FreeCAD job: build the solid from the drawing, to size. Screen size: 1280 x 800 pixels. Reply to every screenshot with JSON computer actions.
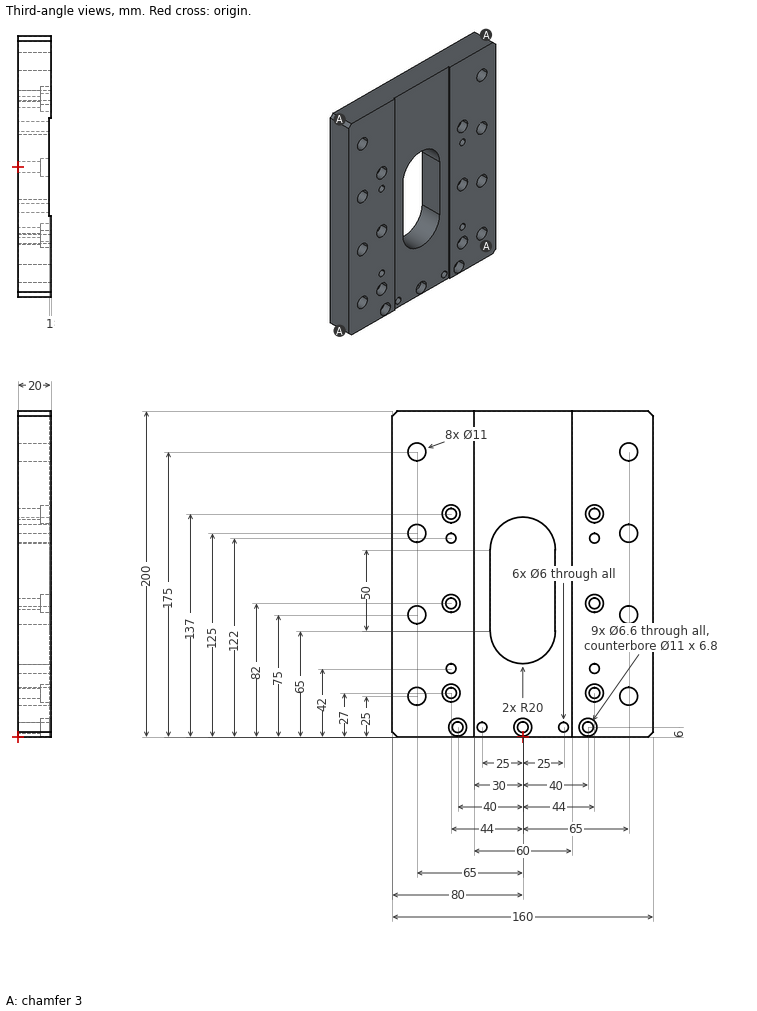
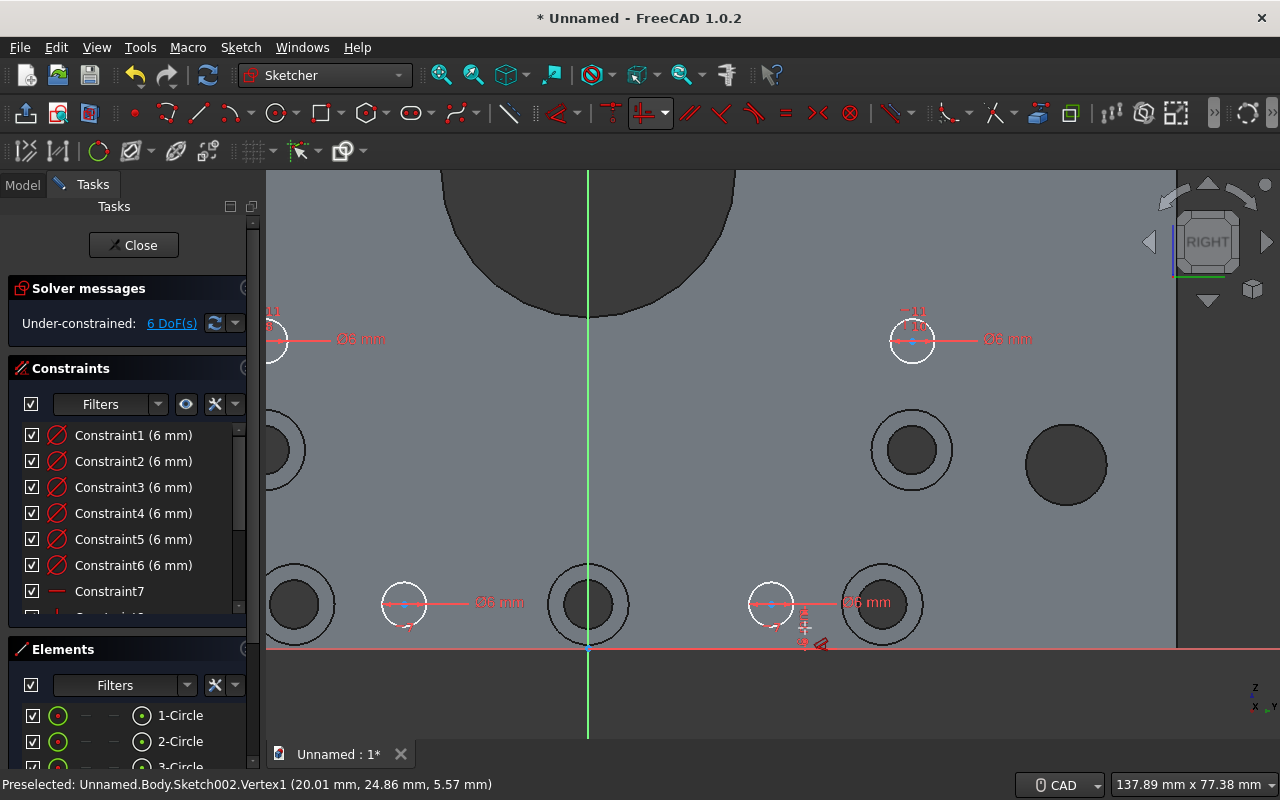
{"action": "left_click", "coordinate": [771, 604]}
{"action": "left_click", "coordinate": [680, 683]}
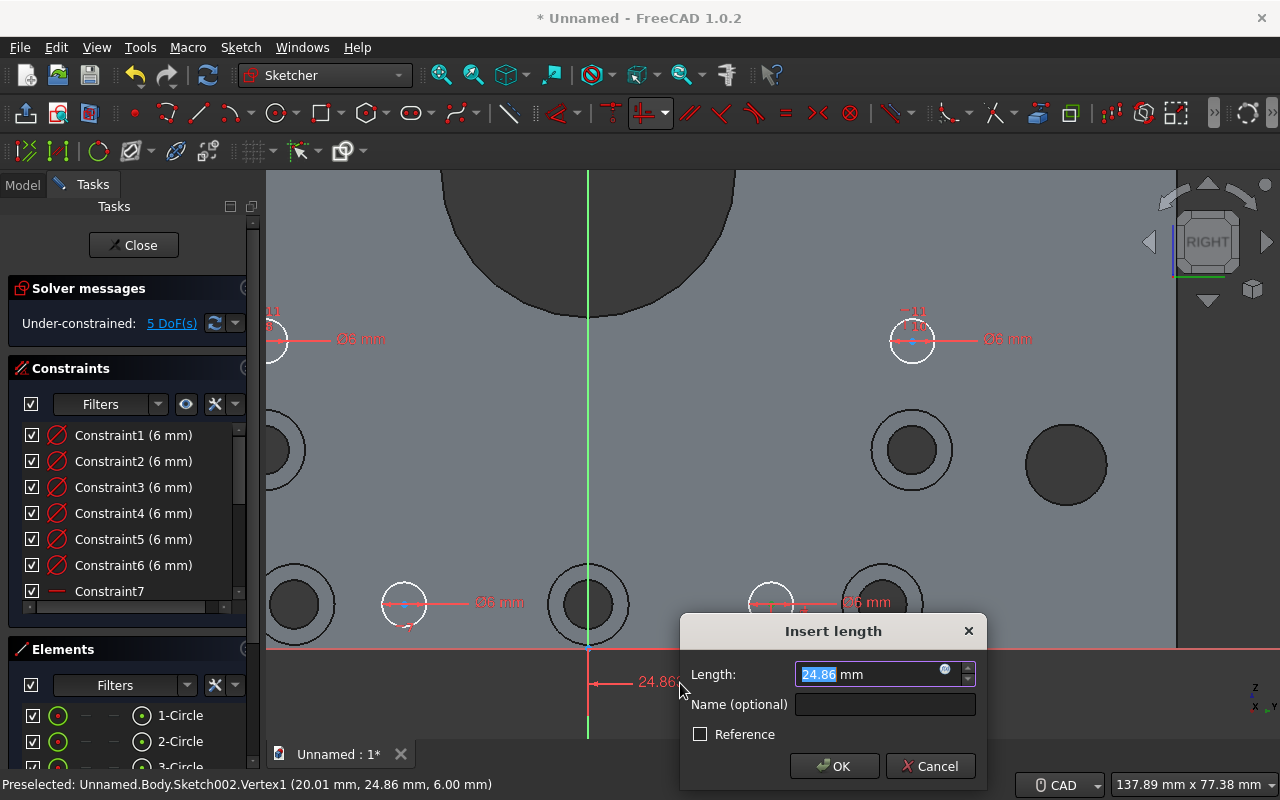
{"action": "type", "text": "25"}
{"action": "key", "text": "Return"}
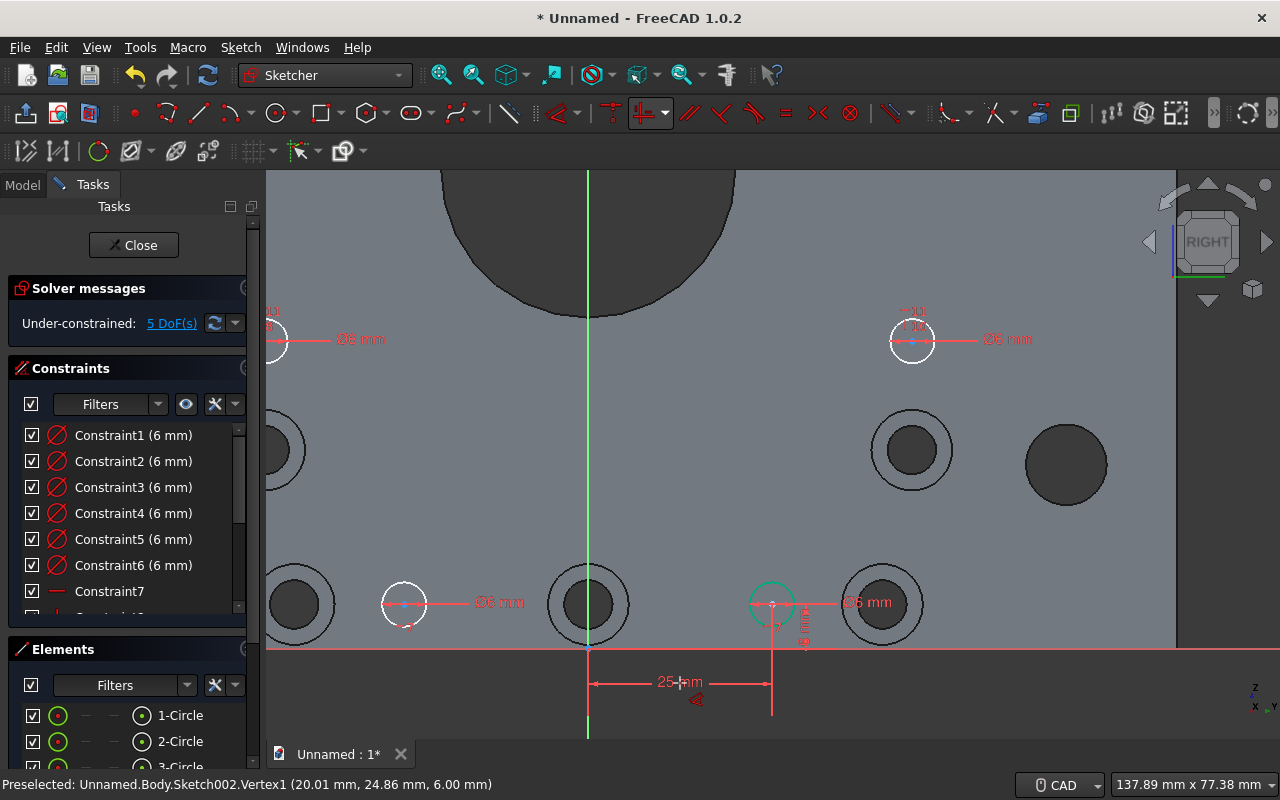
{"action": "left_click", "coordinate": [404, 604]}
{"action": "left_click", "coordinate": [496, 683]}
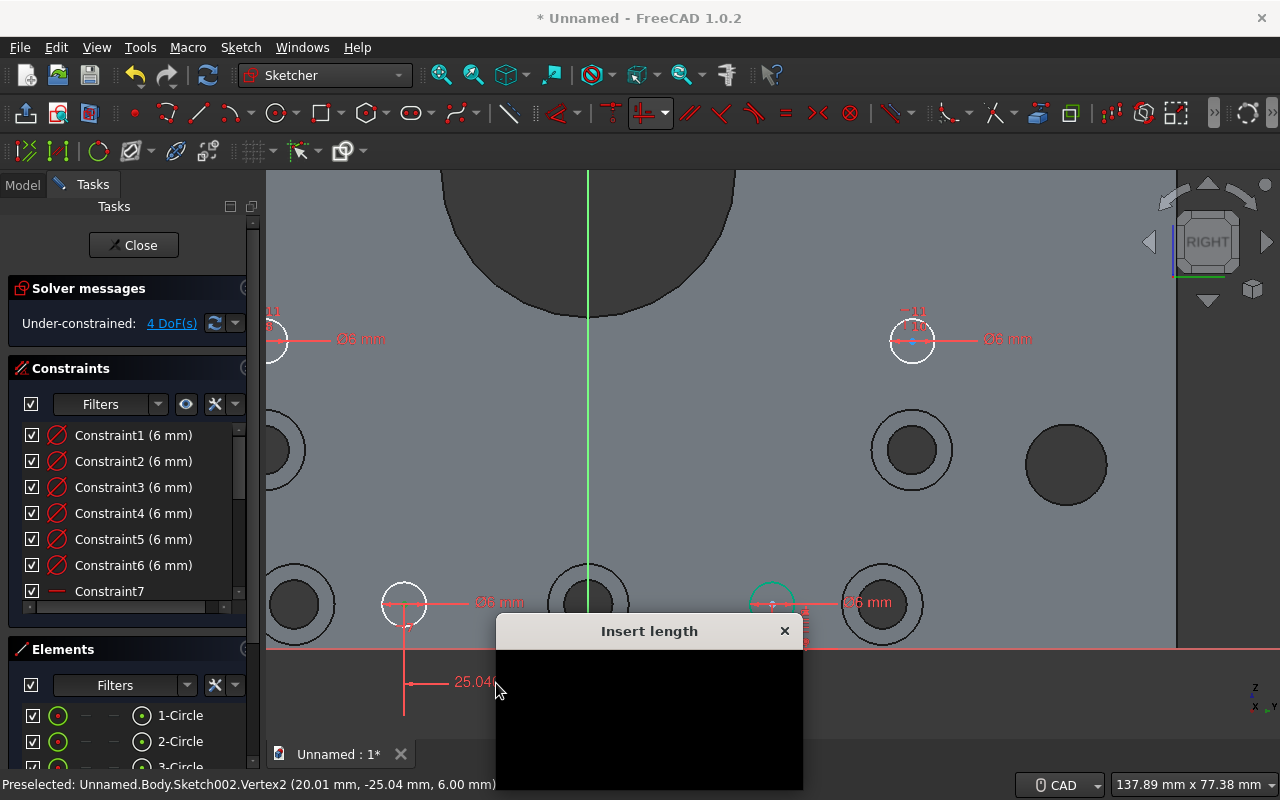
{"action": "type", "text": "25"}
{"action": "key", "text": "Return"}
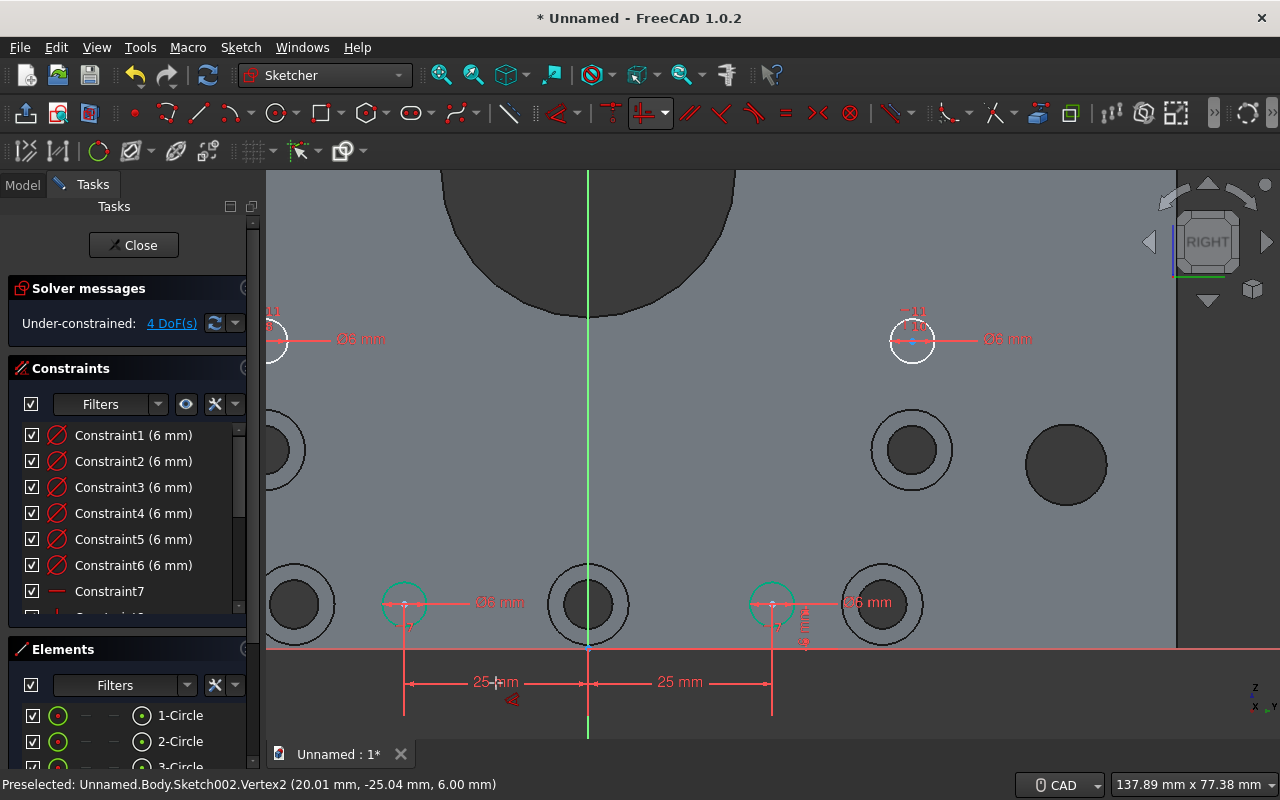
{"action": "scroll", "coordinate": [772, 609], "scroll_direction": "down", "scroll_amount": 5}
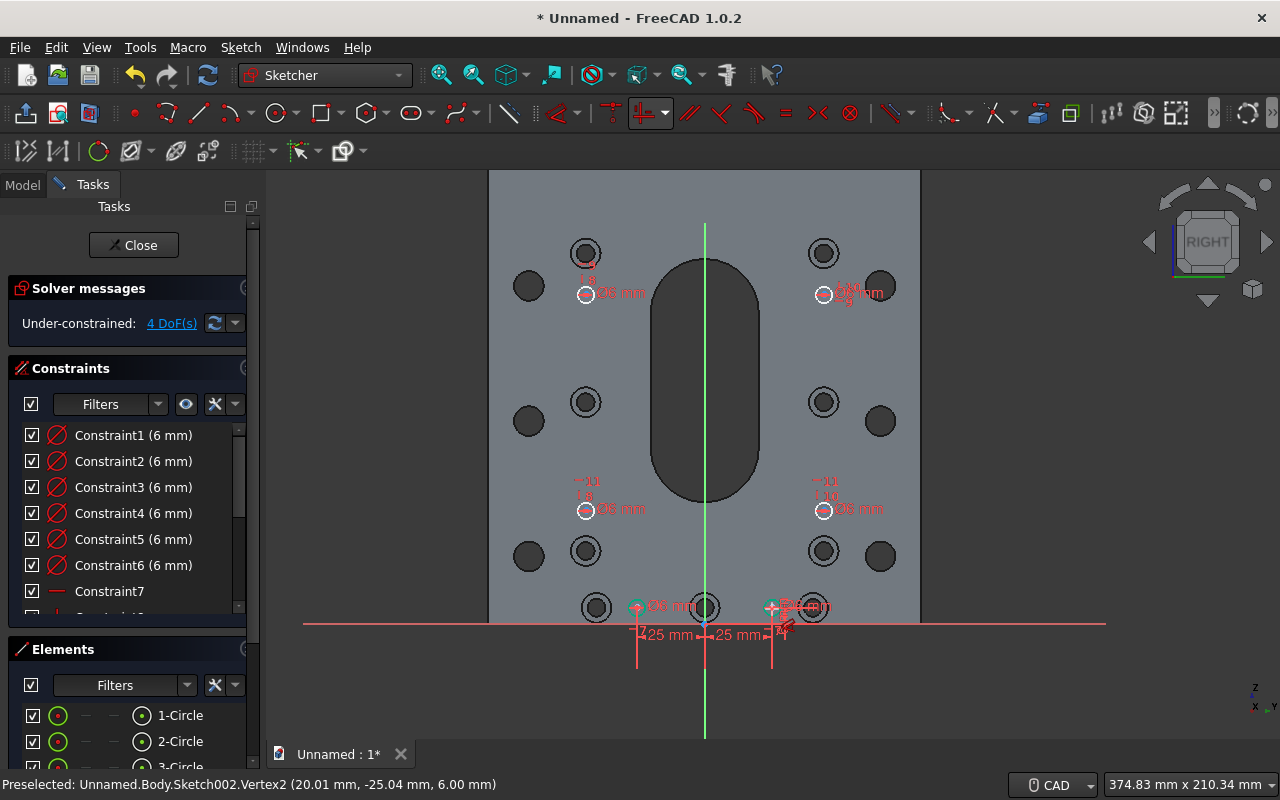
{"action": "left_click", "coordinate": [586, 511]}
{"action": "left_click", "coordinate": [645, 658]}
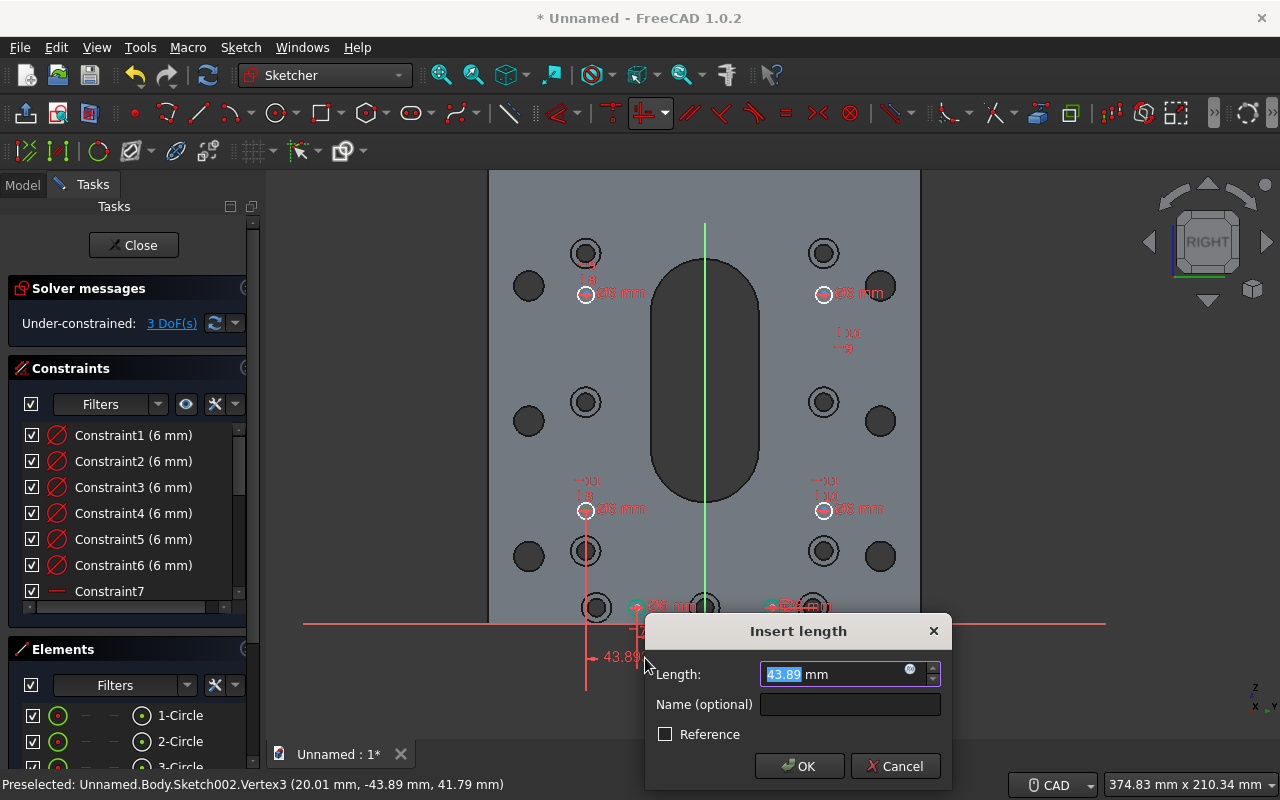
{"action": "type", "text": "44"}
{"action": "key", "text": "Return"}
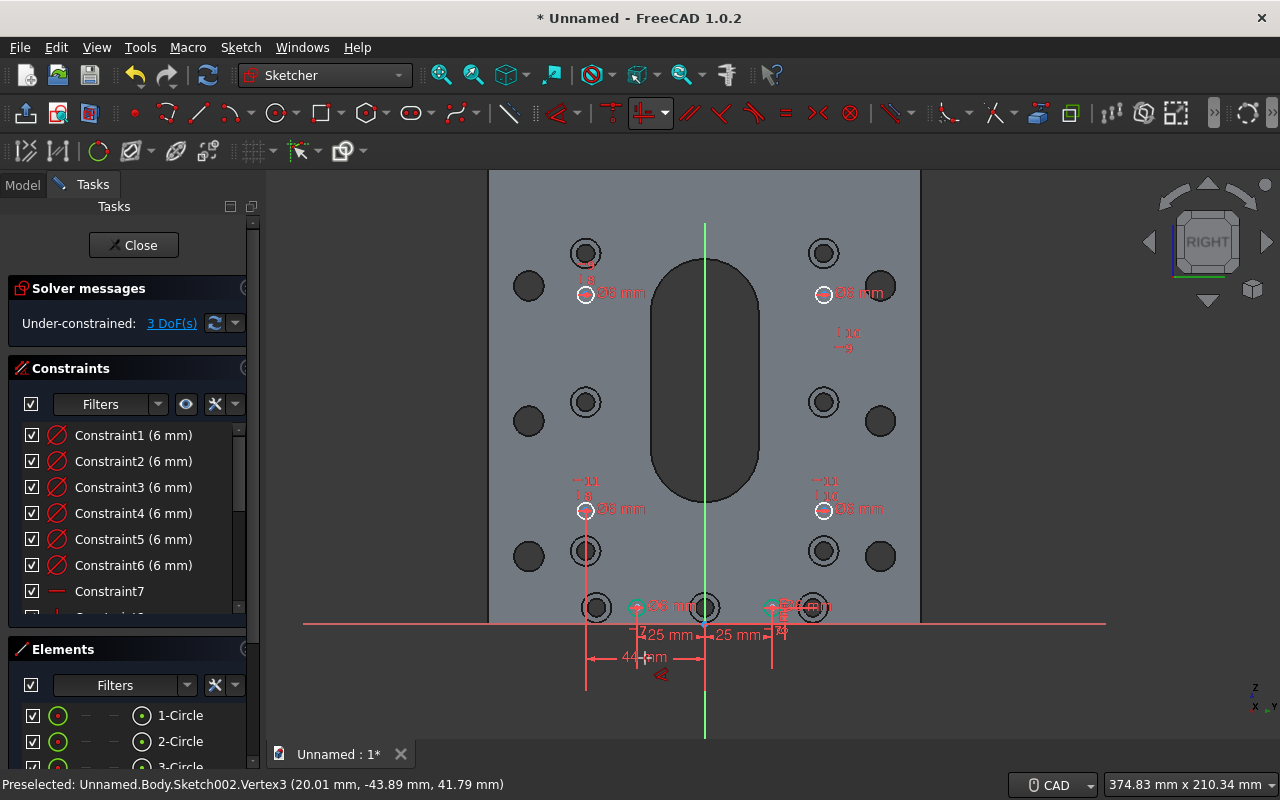
{"action": "left_click", "coordinate": [586, 511]}
{"action": "left_click", "coordinate": [552, 568]}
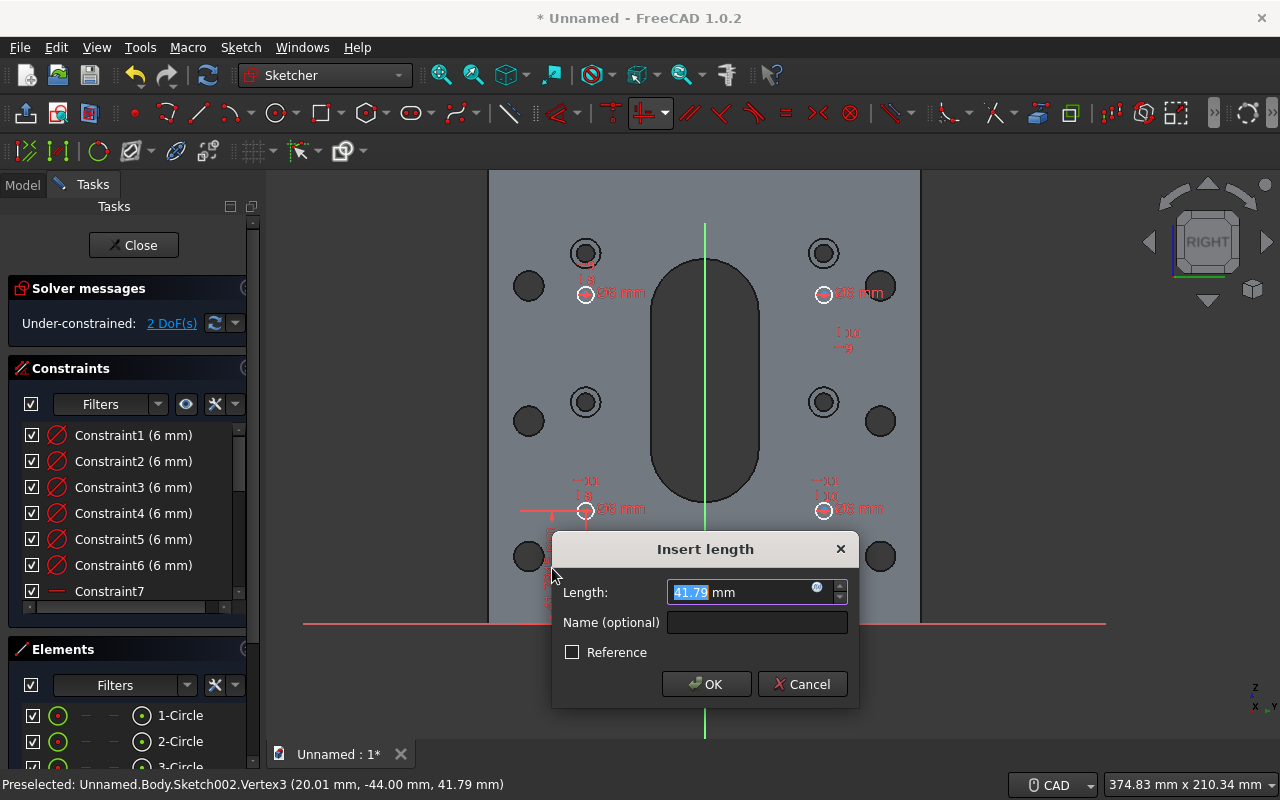
{"action": "type", "text": "42"}
{"action": "key", "text": "Return"}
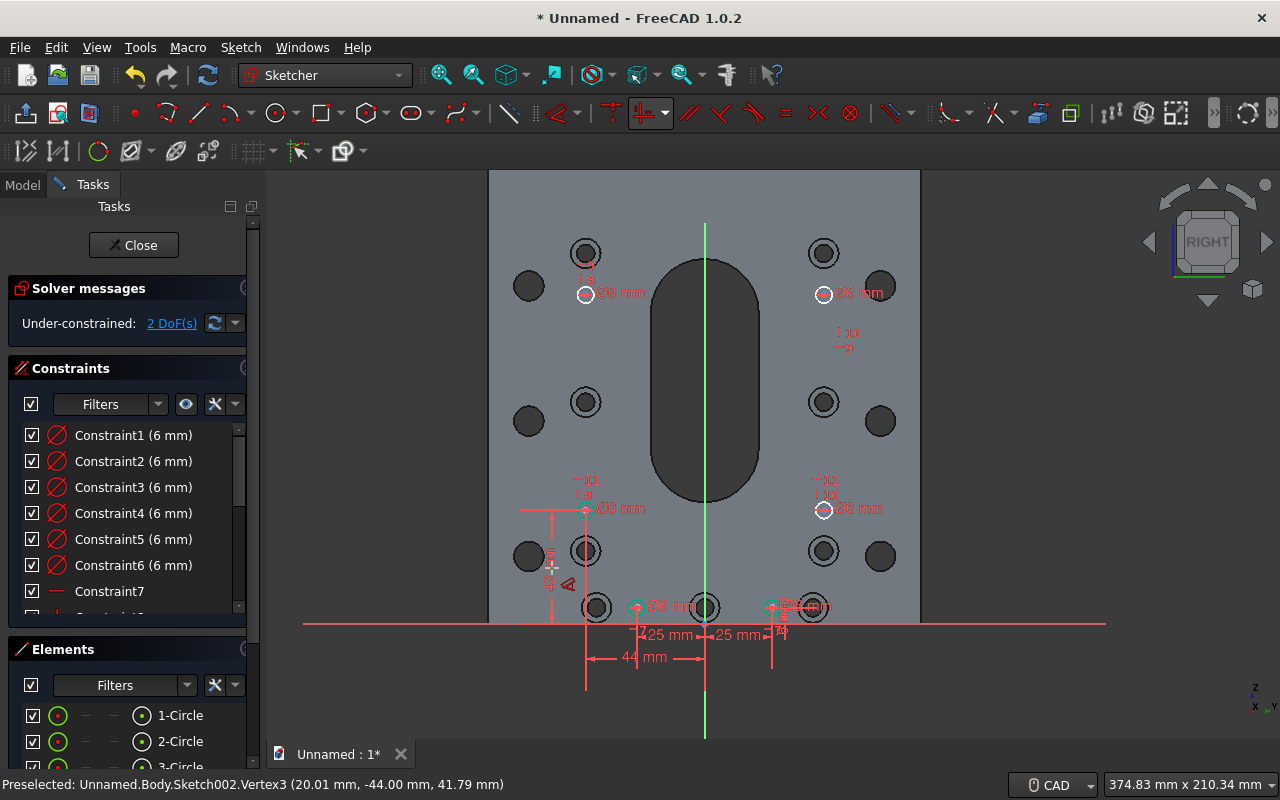
{"action": "left_click", "coordinate": [824, 295]}
{"action": "left_click", "coordinate": [764, 658]}